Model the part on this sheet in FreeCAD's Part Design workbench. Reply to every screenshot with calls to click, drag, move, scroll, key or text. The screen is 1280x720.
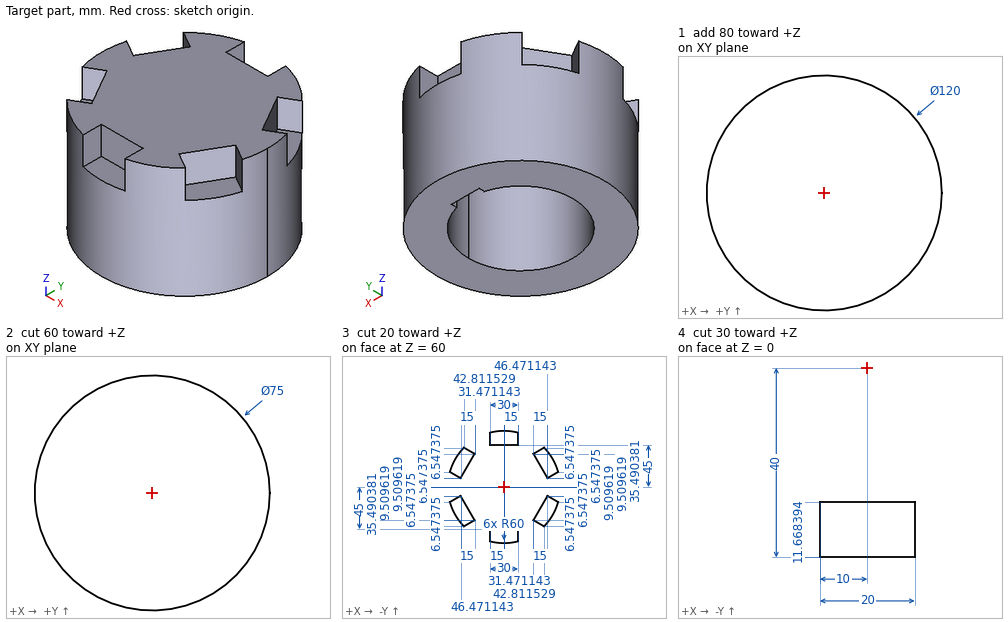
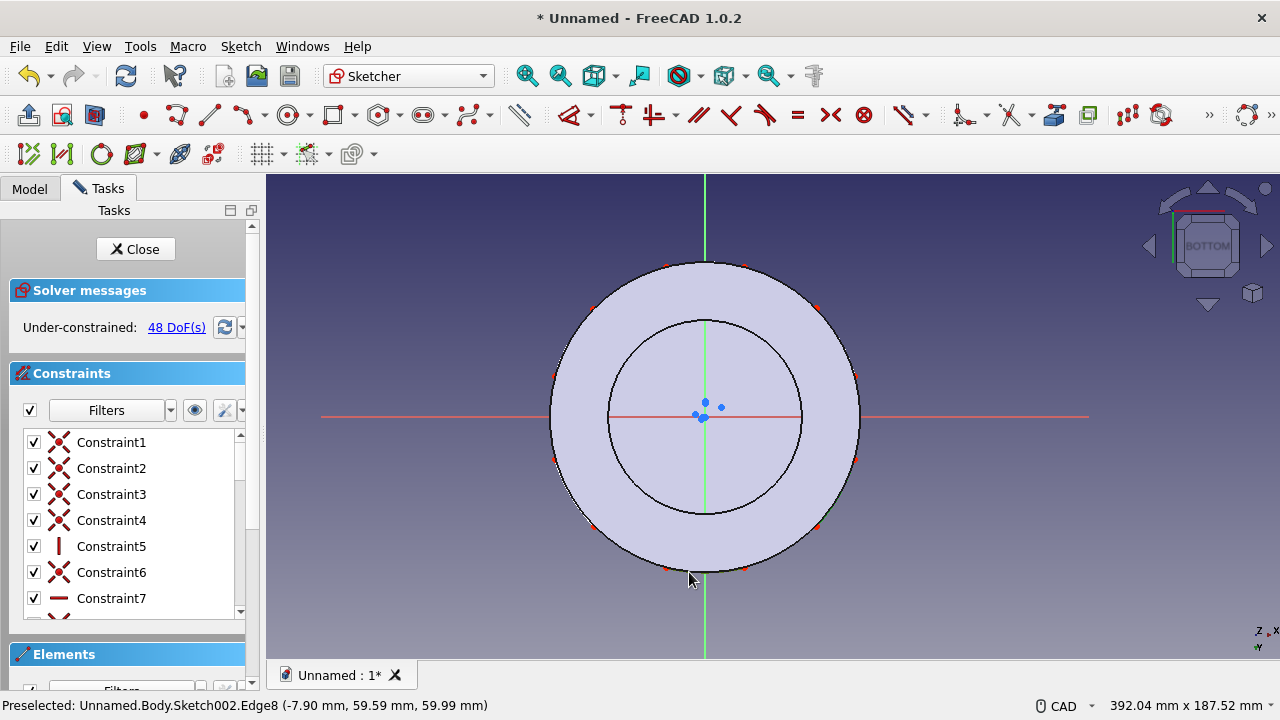
click(621, 116)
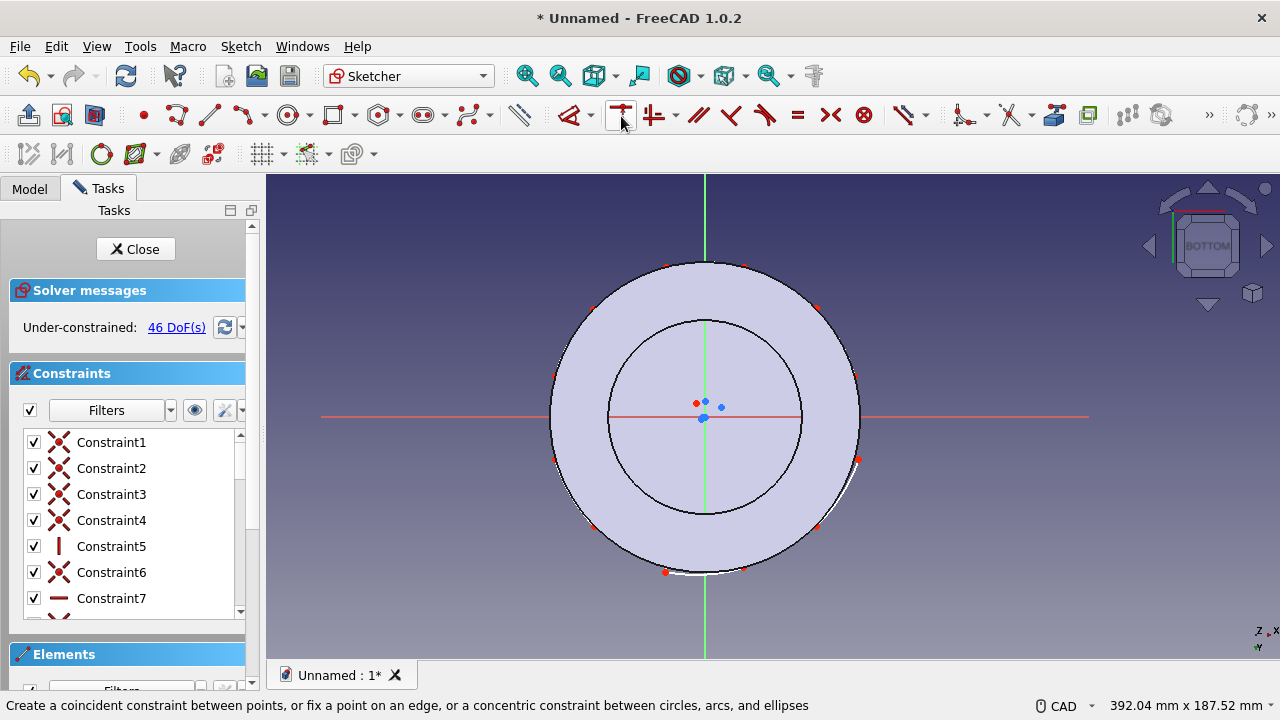
click(832, 509)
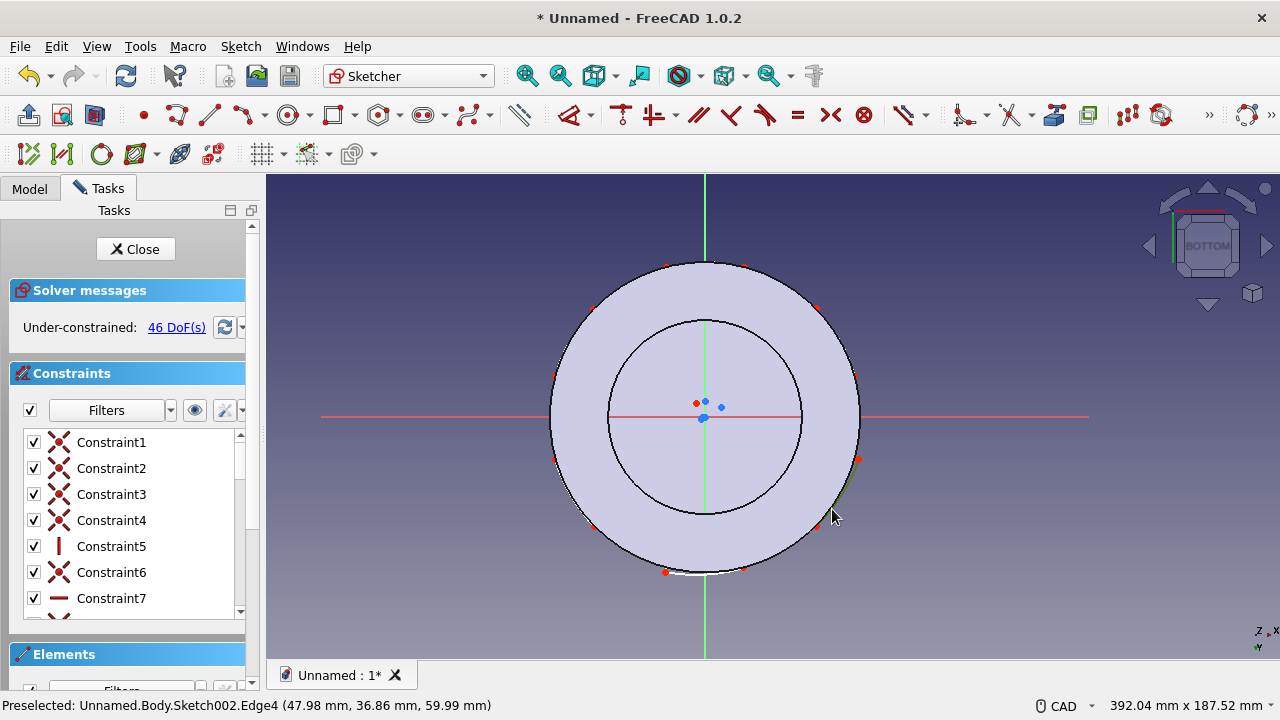
click(847, 355)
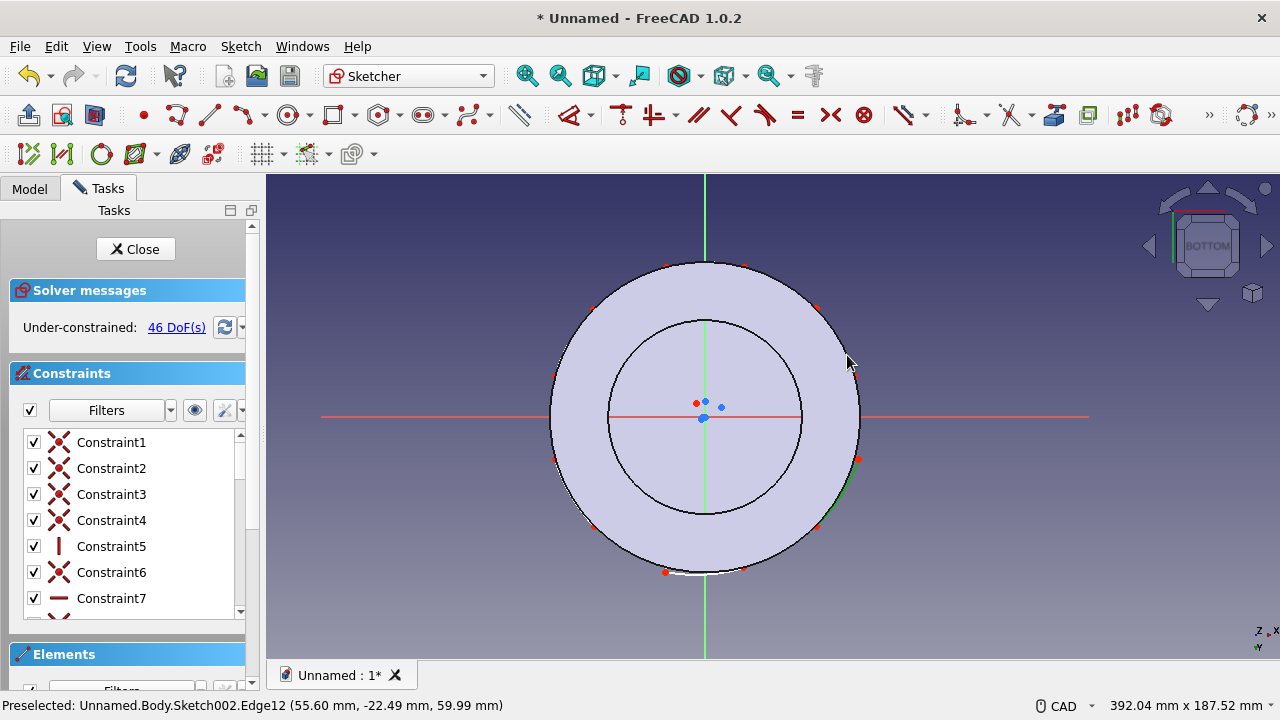
click(621, 116)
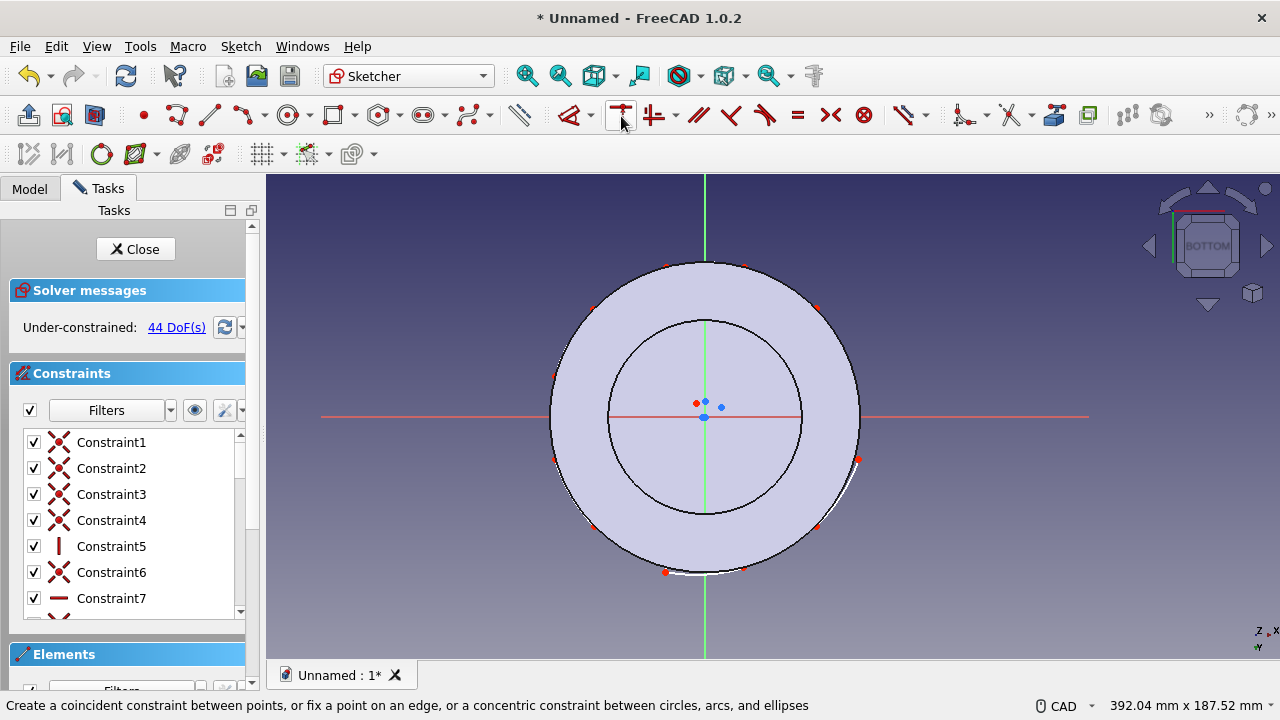
click(832, 509)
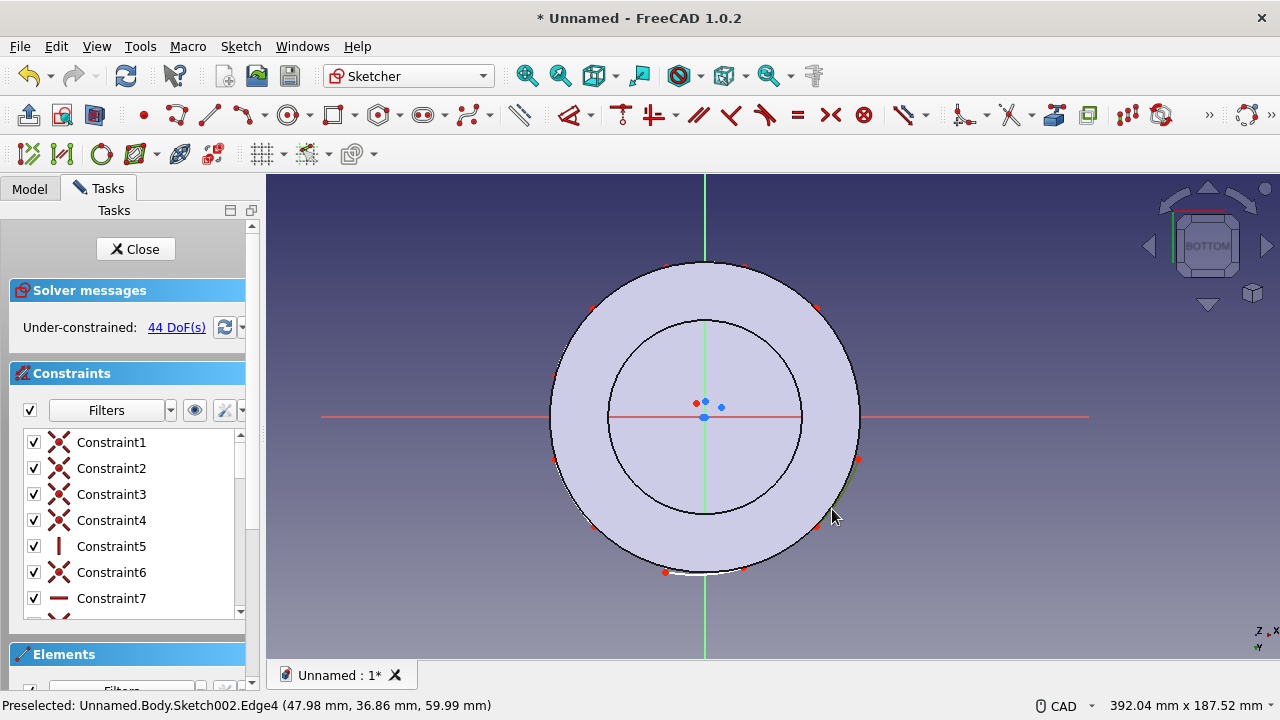
click(721, 263)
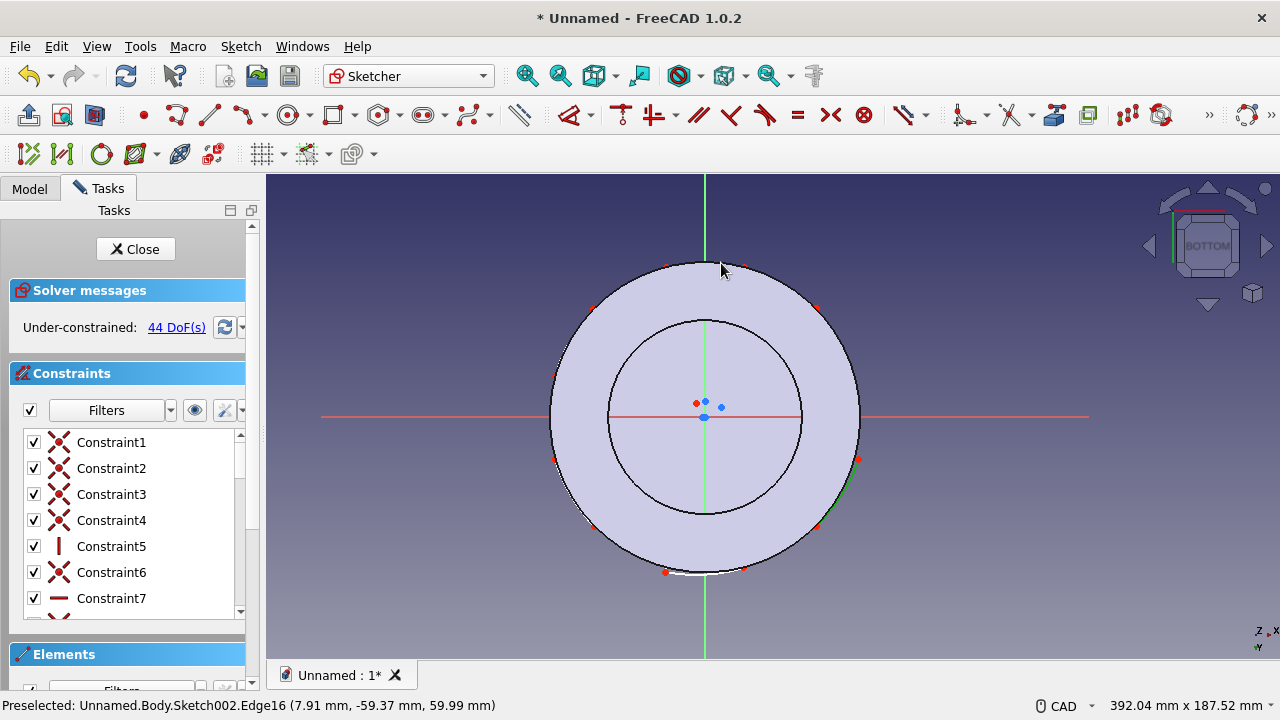
click(621, 116)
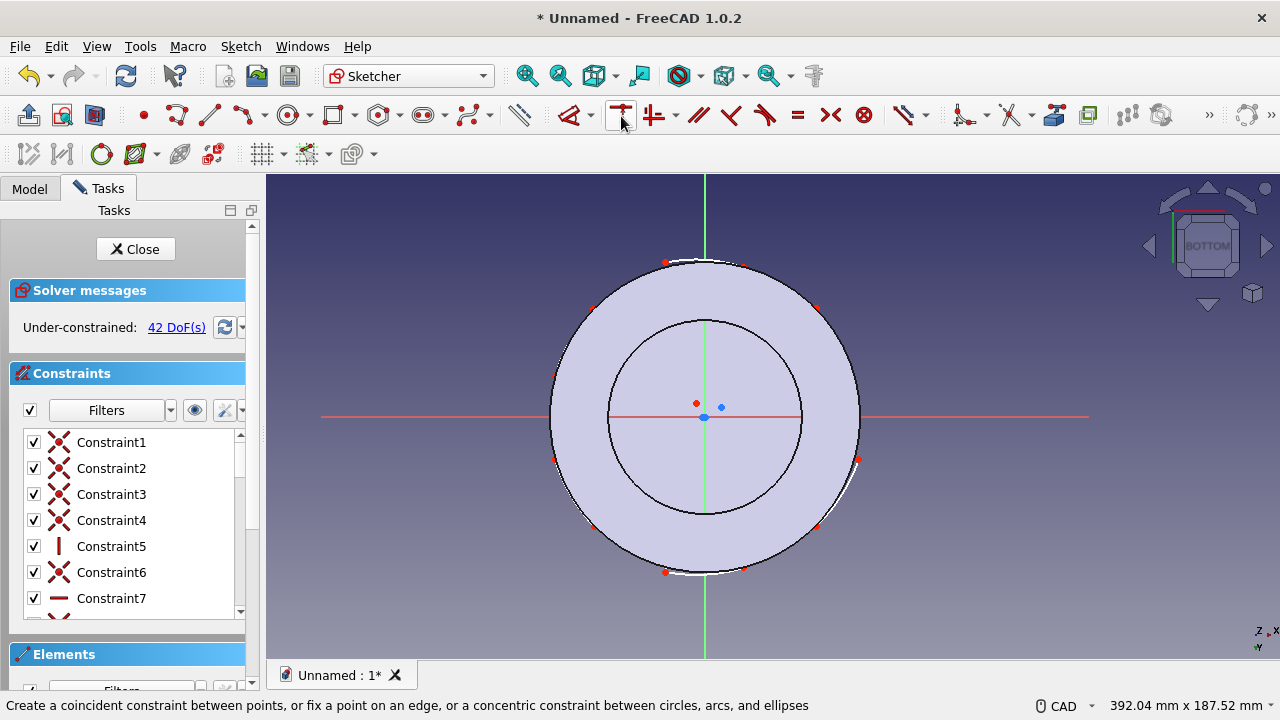
click(832, 509)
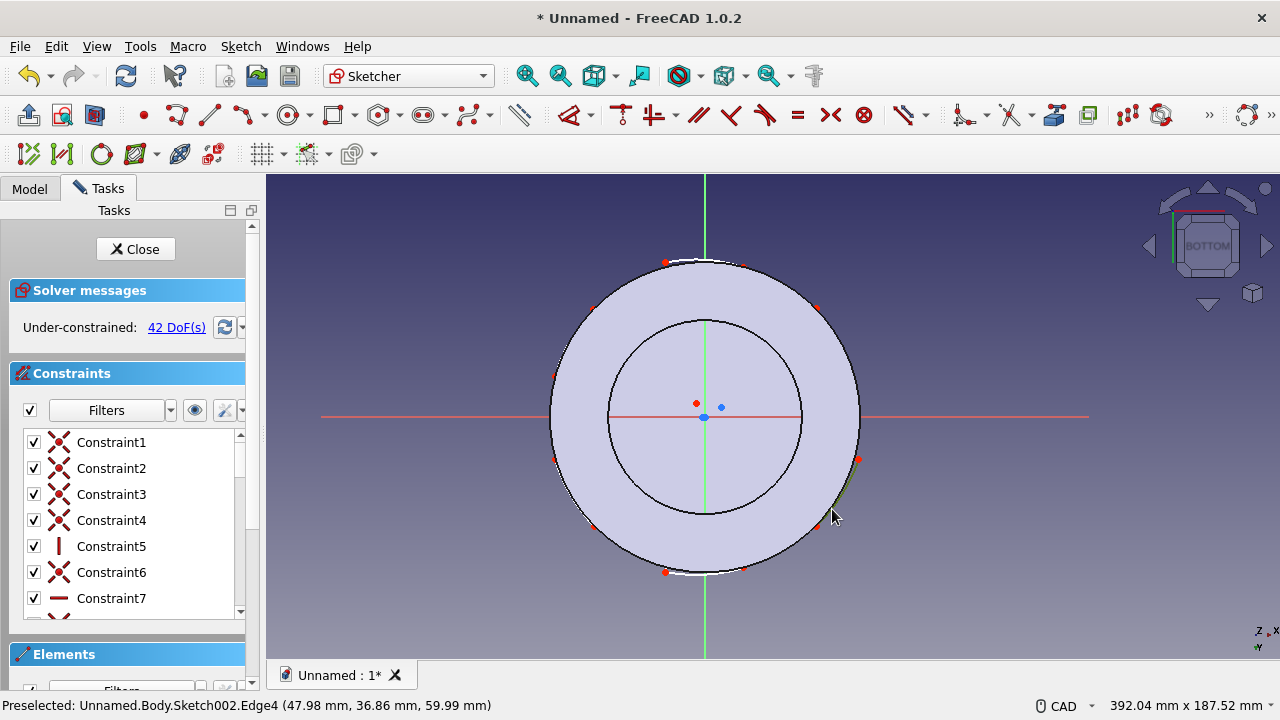
click(579, 328)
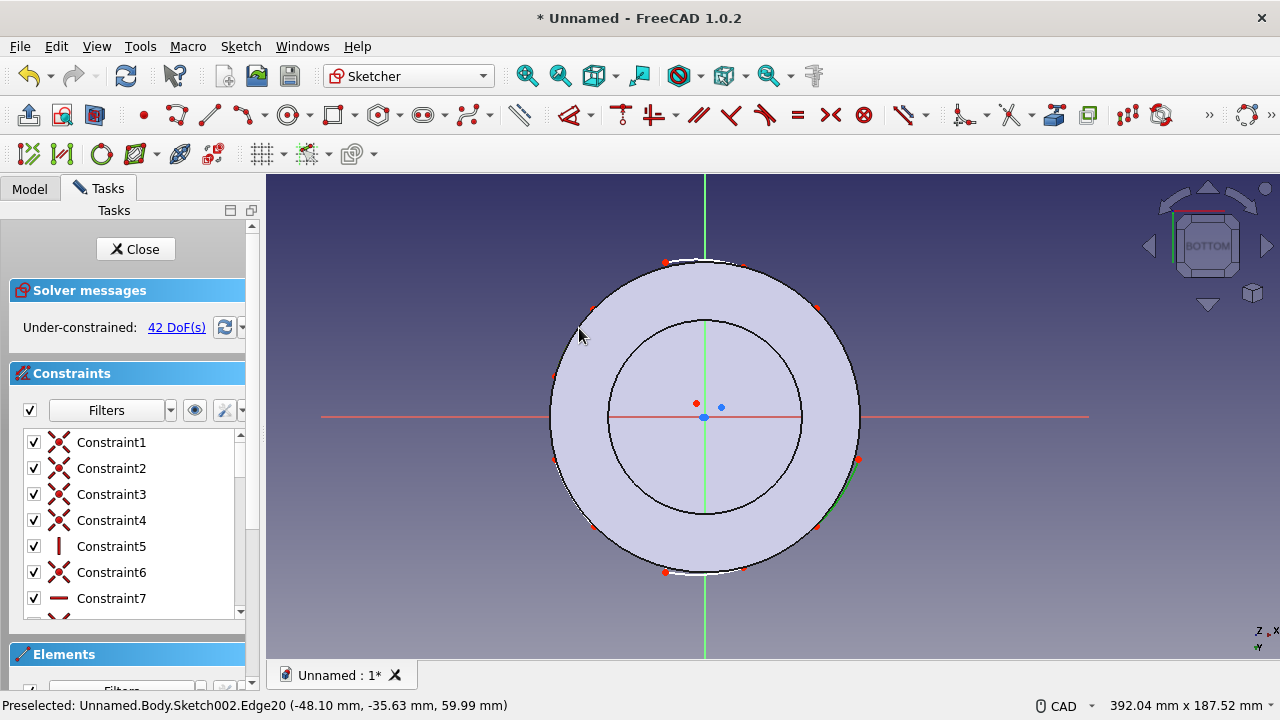
click(621, 116)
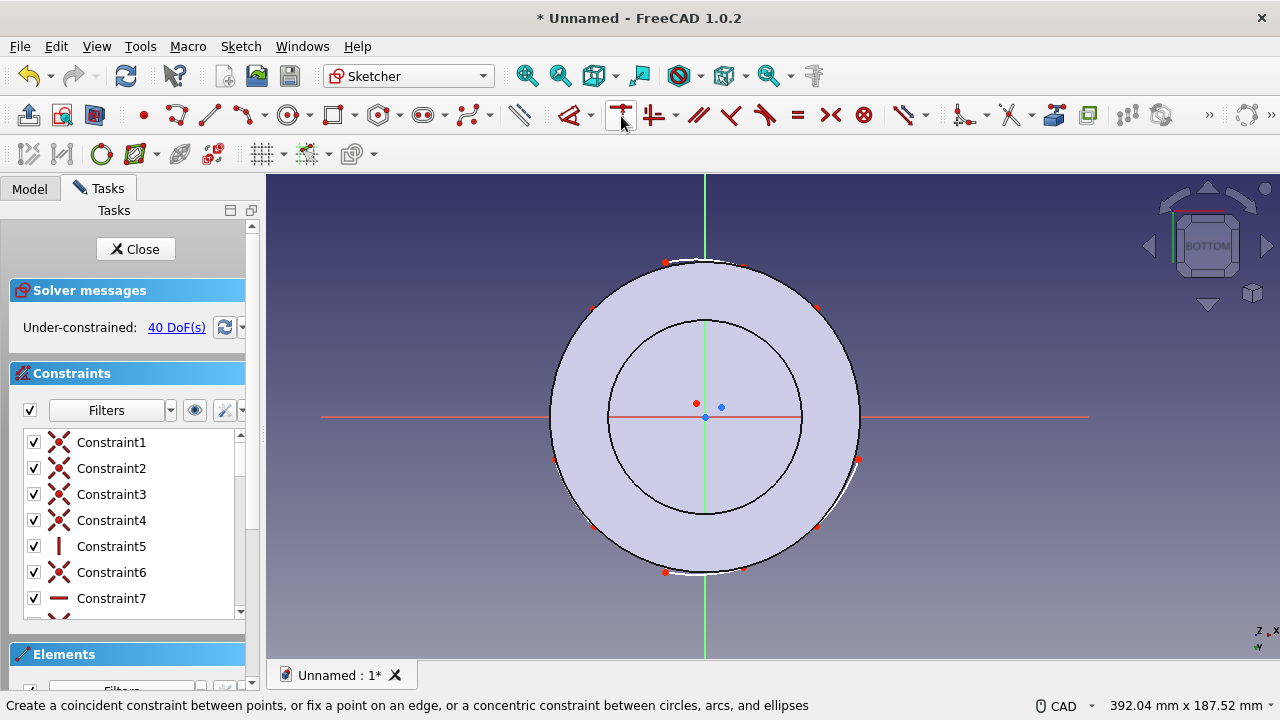
click(832, 509)